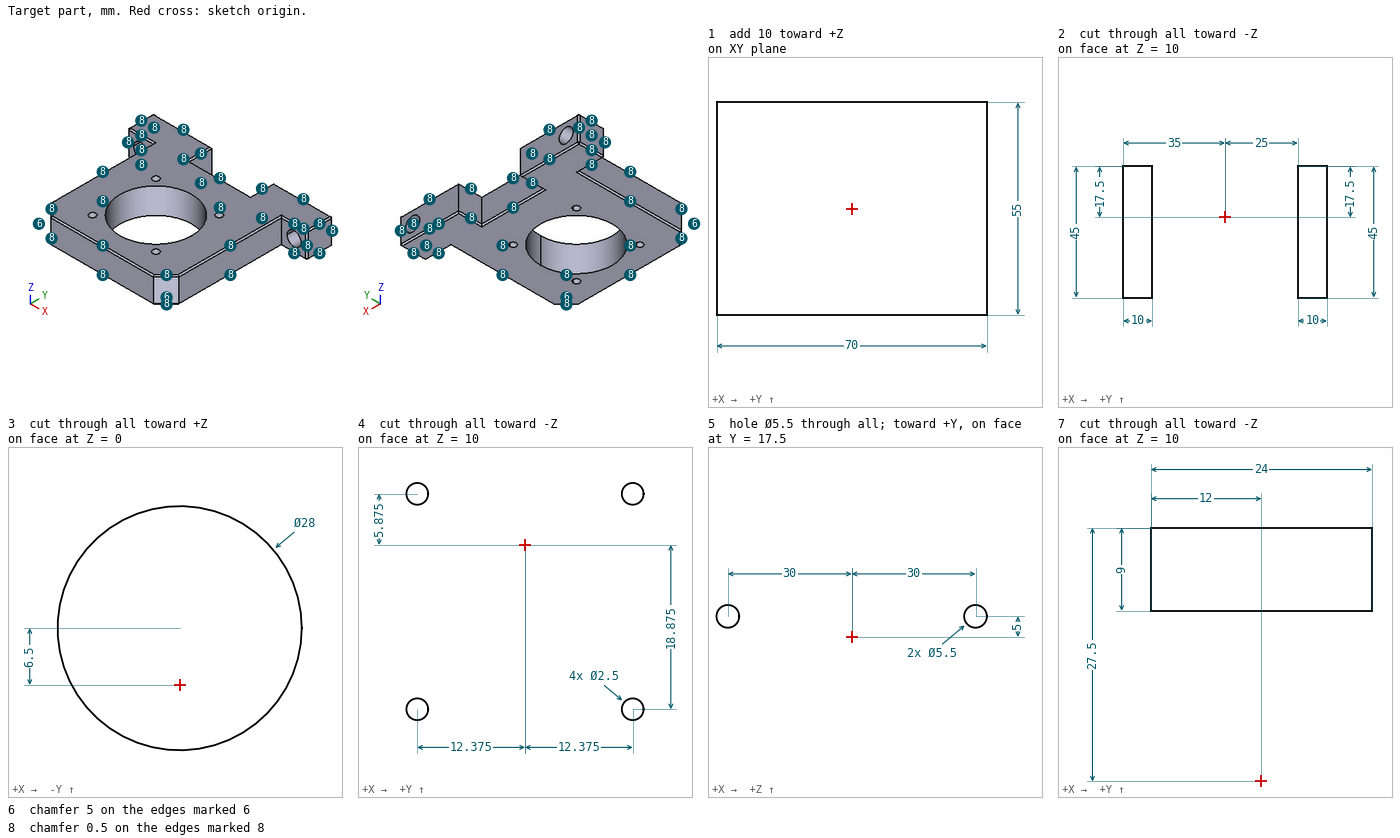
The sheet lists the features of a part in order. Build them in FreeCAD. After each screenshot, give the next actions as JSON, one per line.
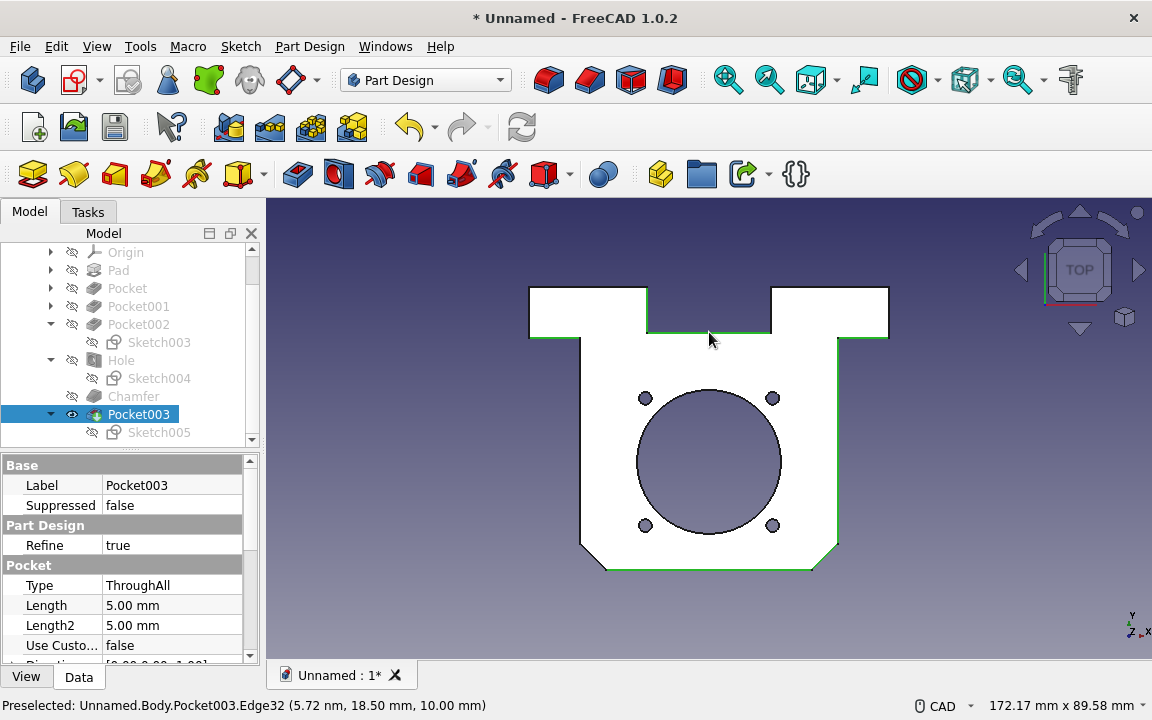
{"action": "left_click", "coordinate": [771, 309], "text": "ctrl"}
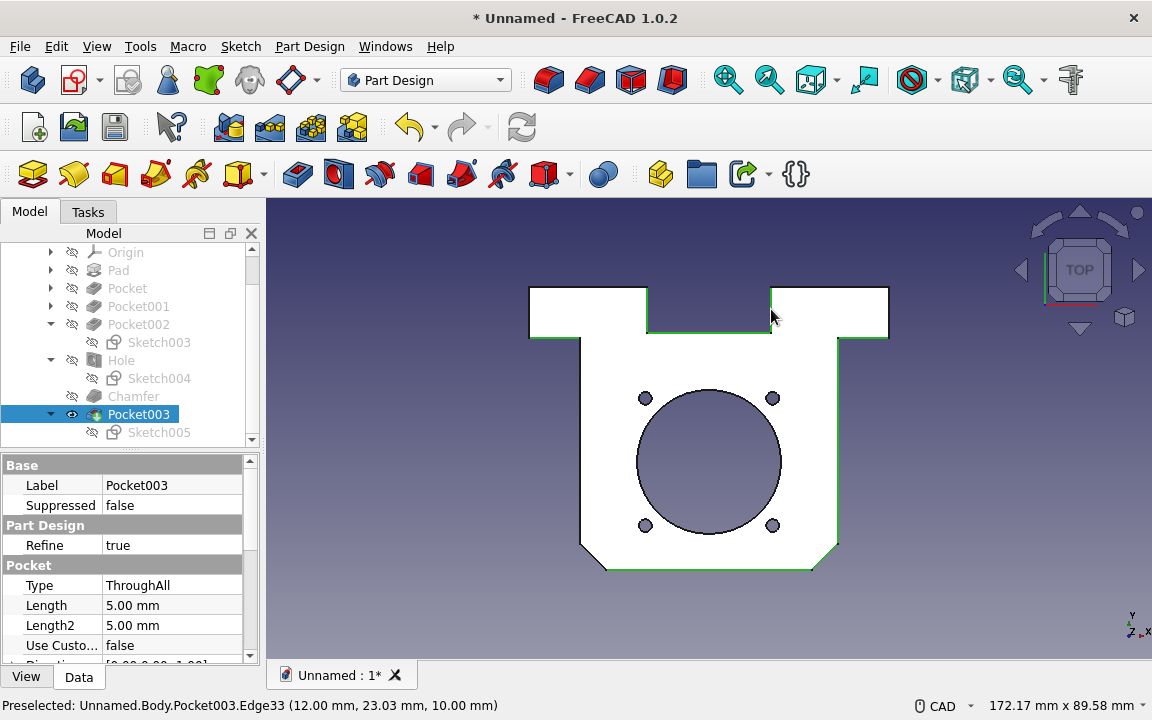
{"action": "left_click", "coordinate": [830, 286], "text": "ctrl"}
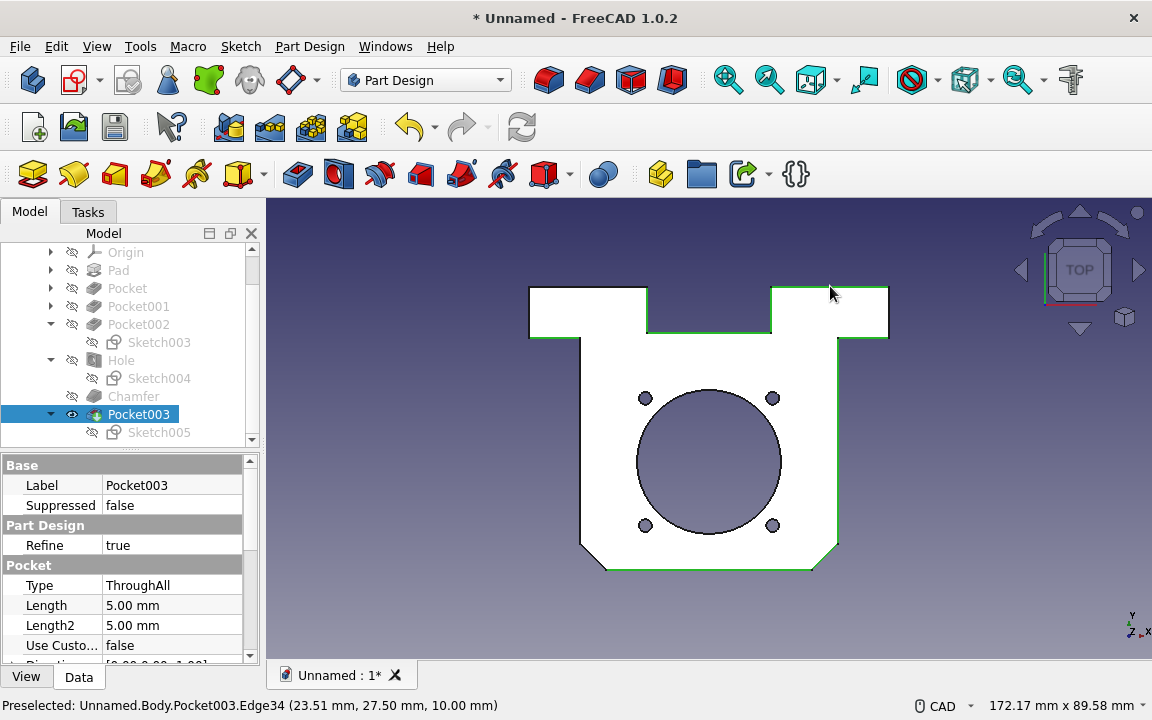
{"action": "left_click", "coordinate": [580, 440], "text": "ctrl"}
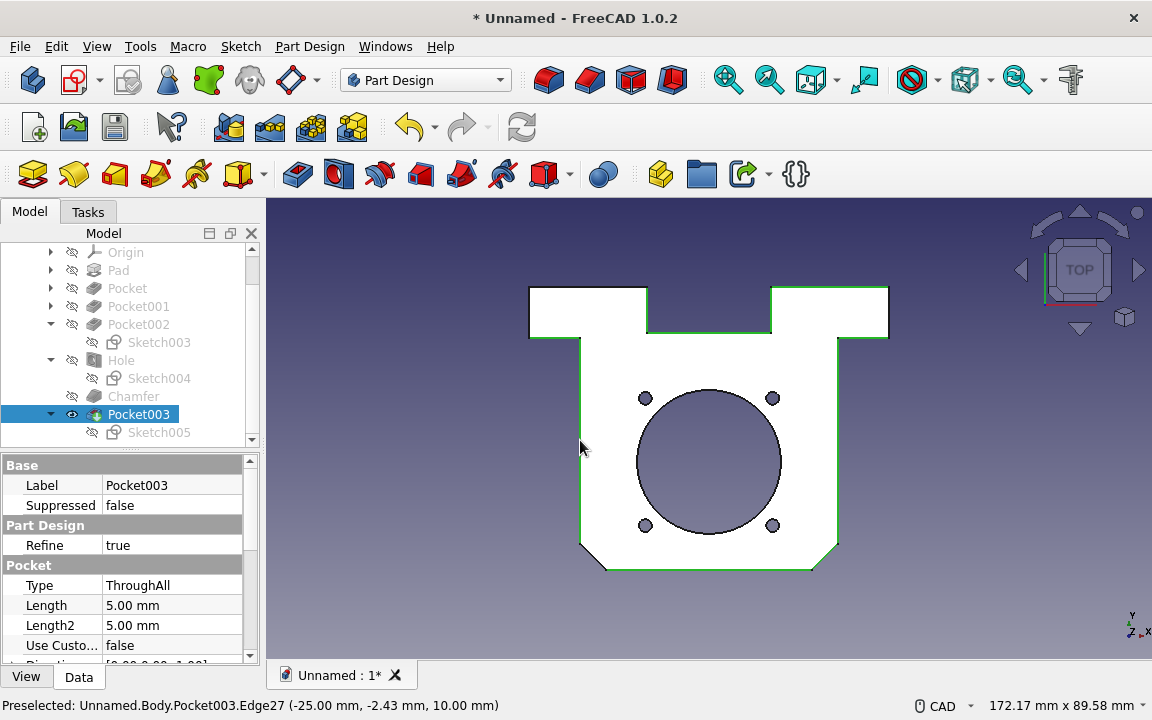
{"action": "left_click", "coordinate": [593, 556], "text": "ctrl"}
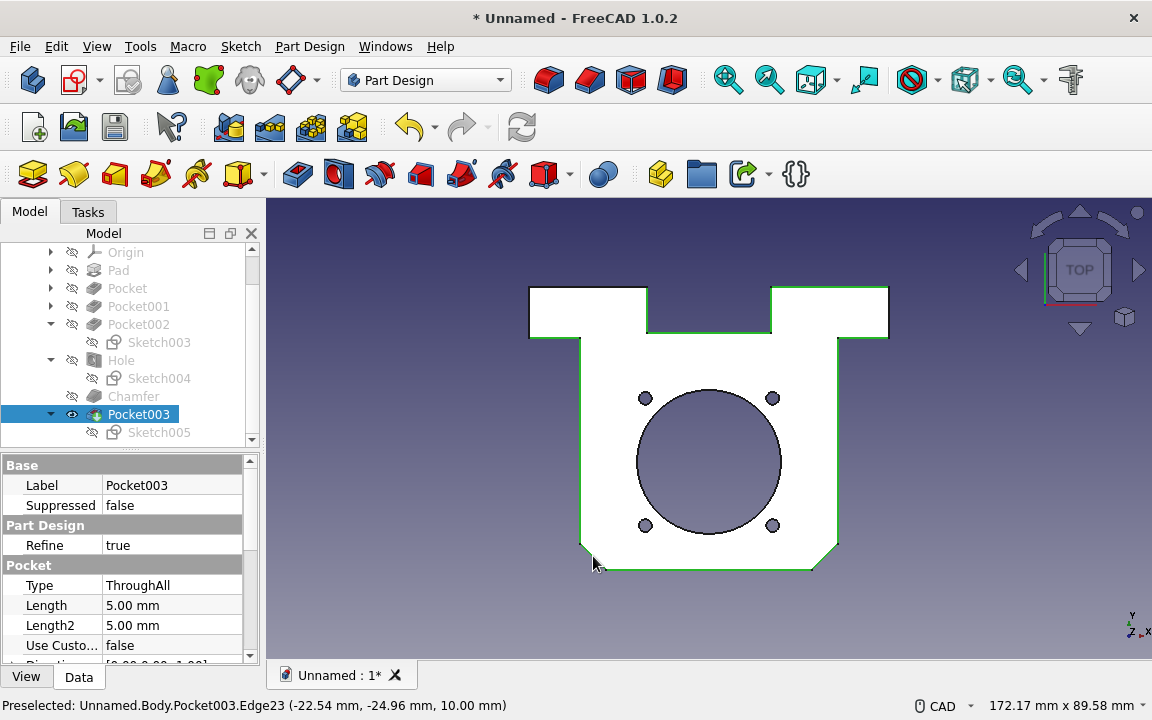
{"action": "left_click", "coordinate": [588, 286], "text": "ctrl"}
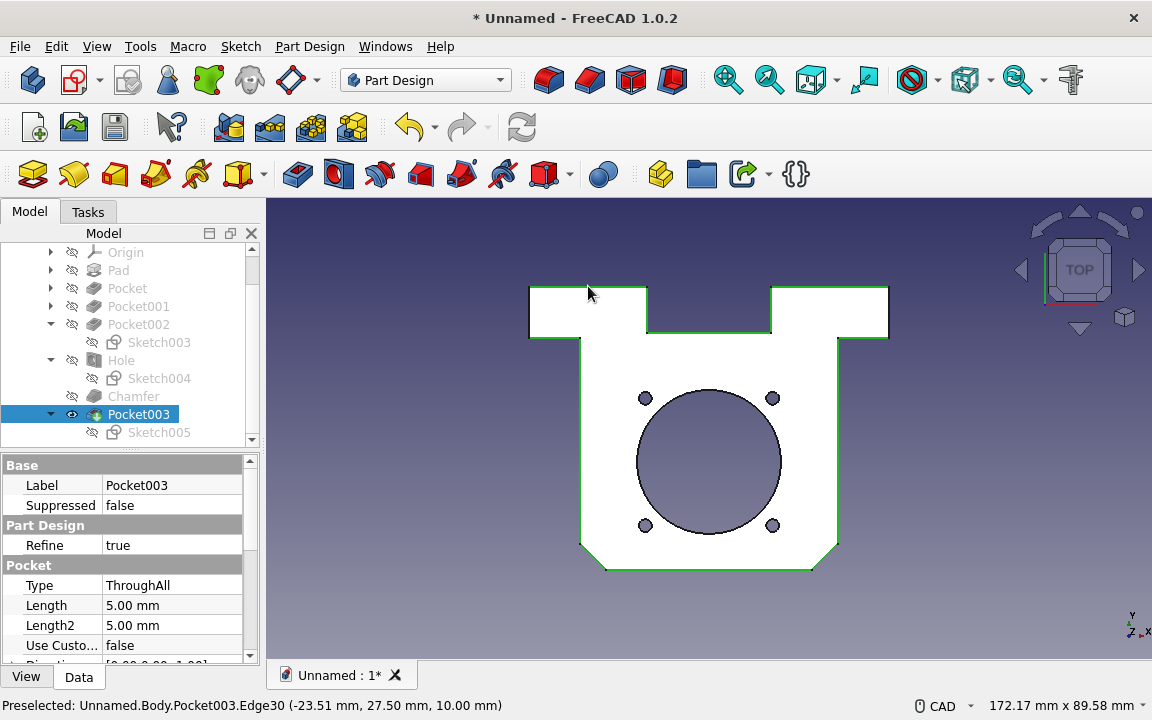
{"action": "key", "text": "0"}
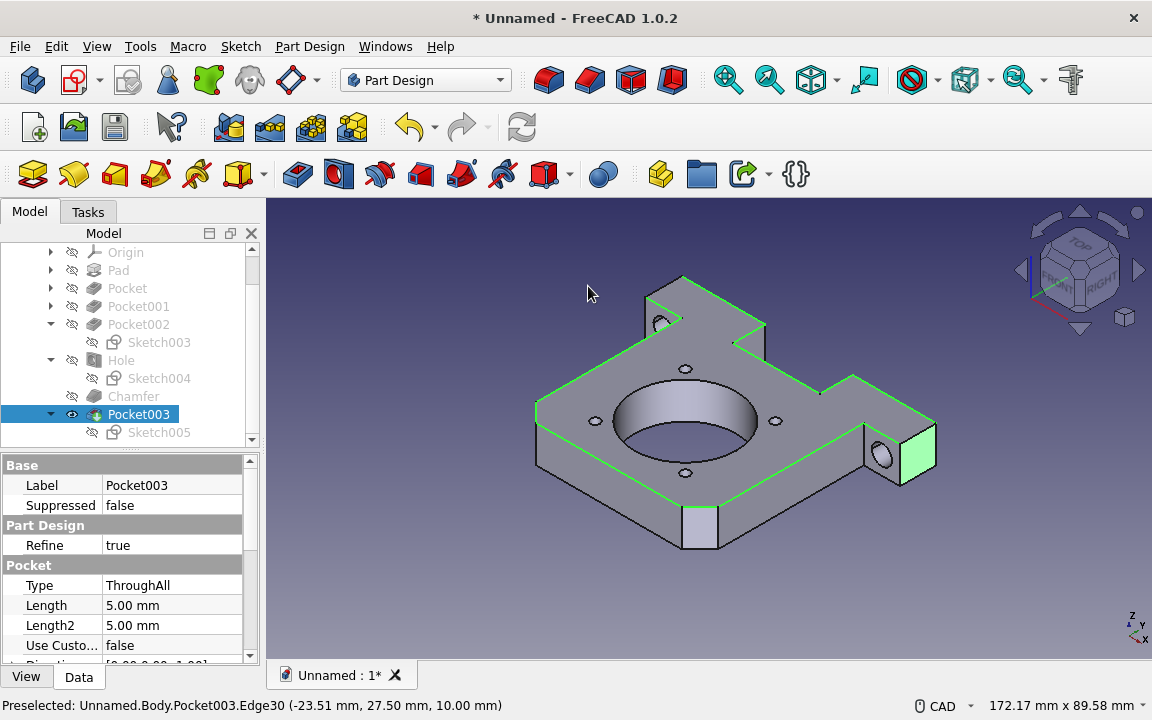
{"action": "key", "text": "1"}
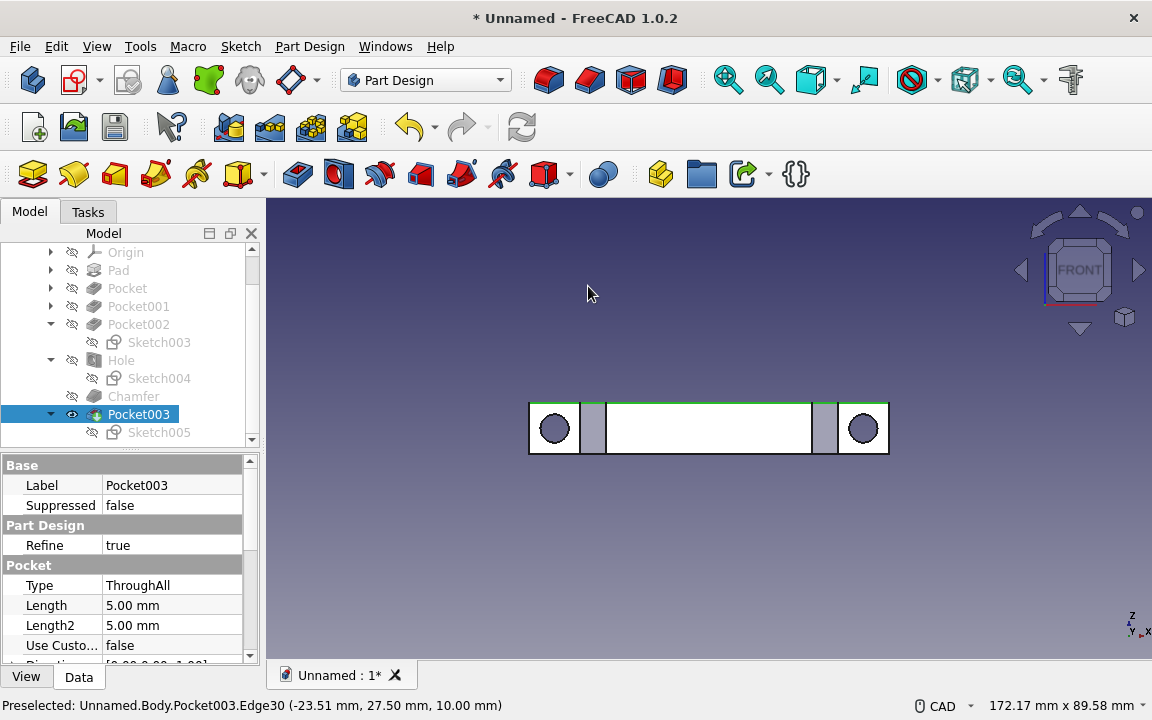
{"action": "left_click", "coordinate": [729, 80]}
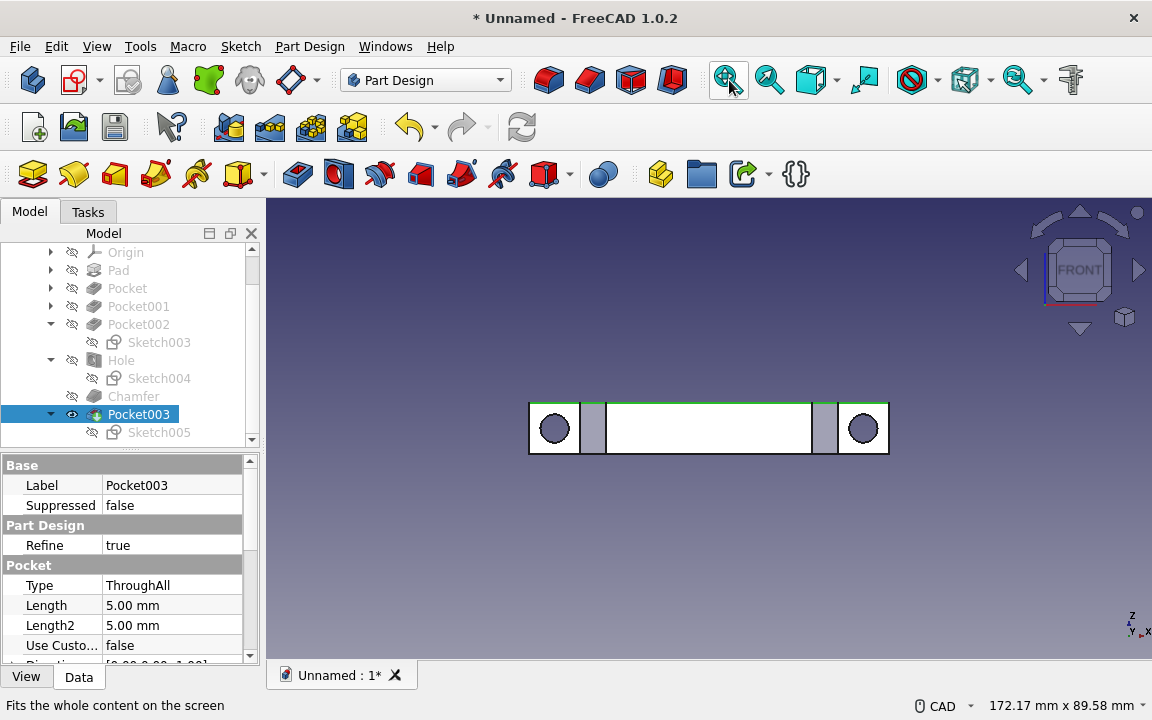
{"action": "left_click", "coordinate": [555, 453], "text": "ctrl"}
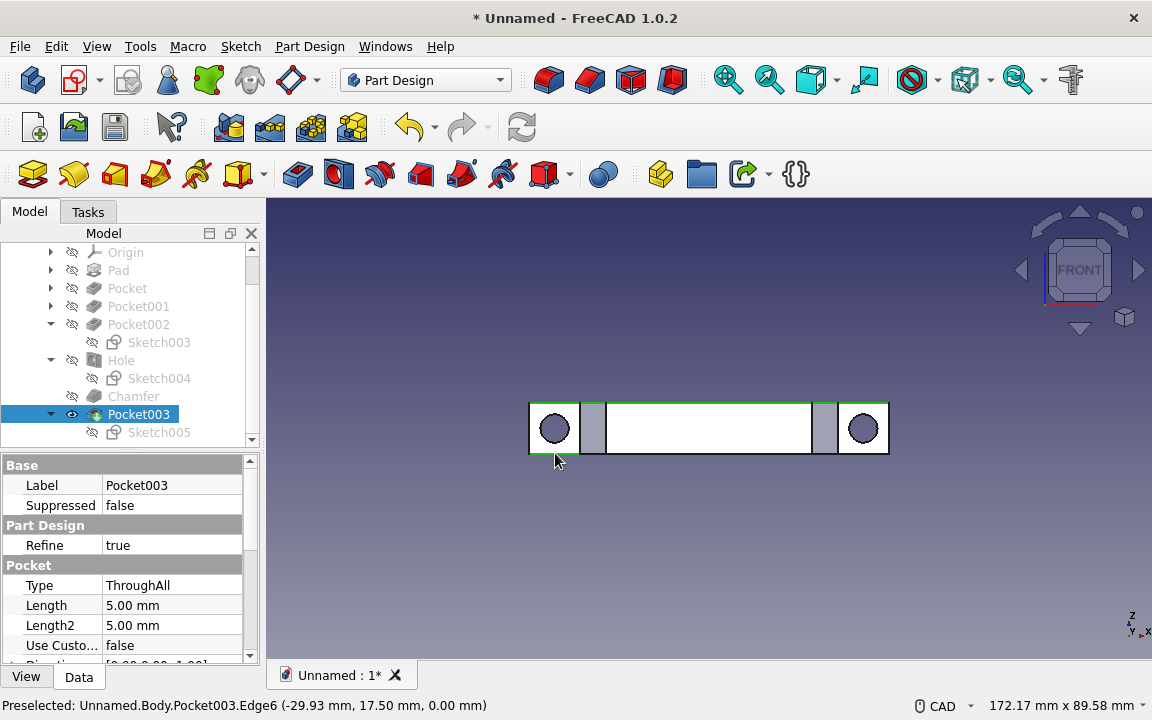
{"action": "left_click", "coordinate": [863, 453], "text": "ctrl"}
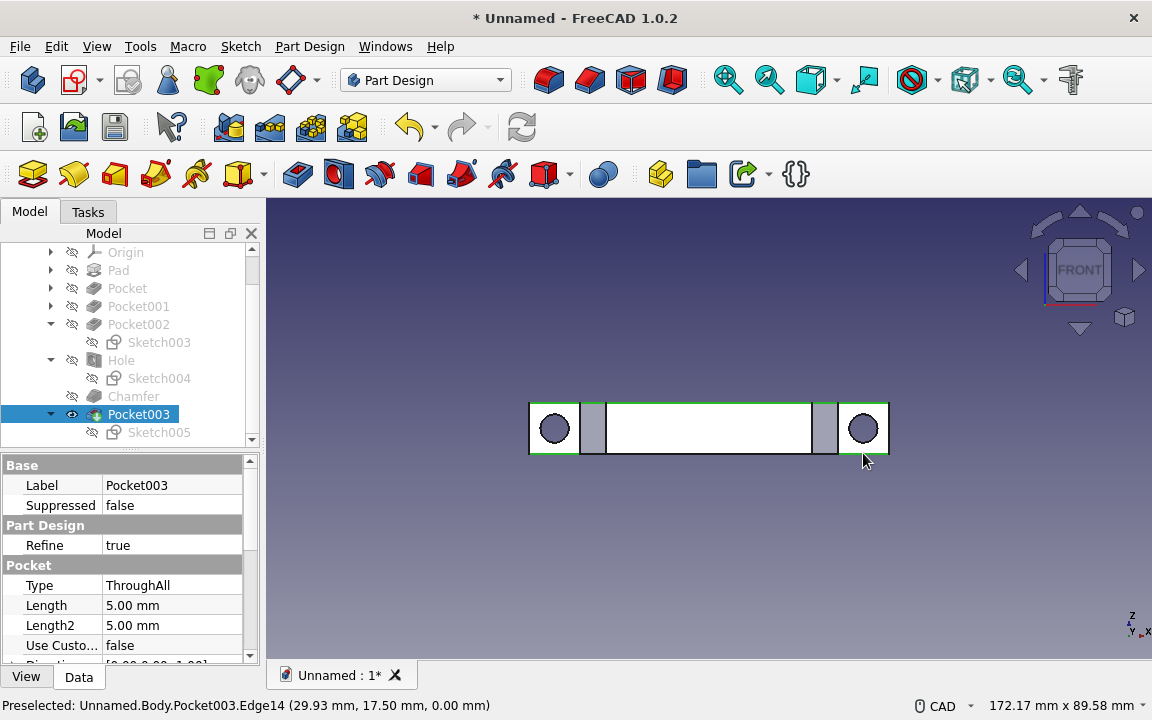
{"action": "left_click", "coordinate": [709, 453], "text": "ctrl"}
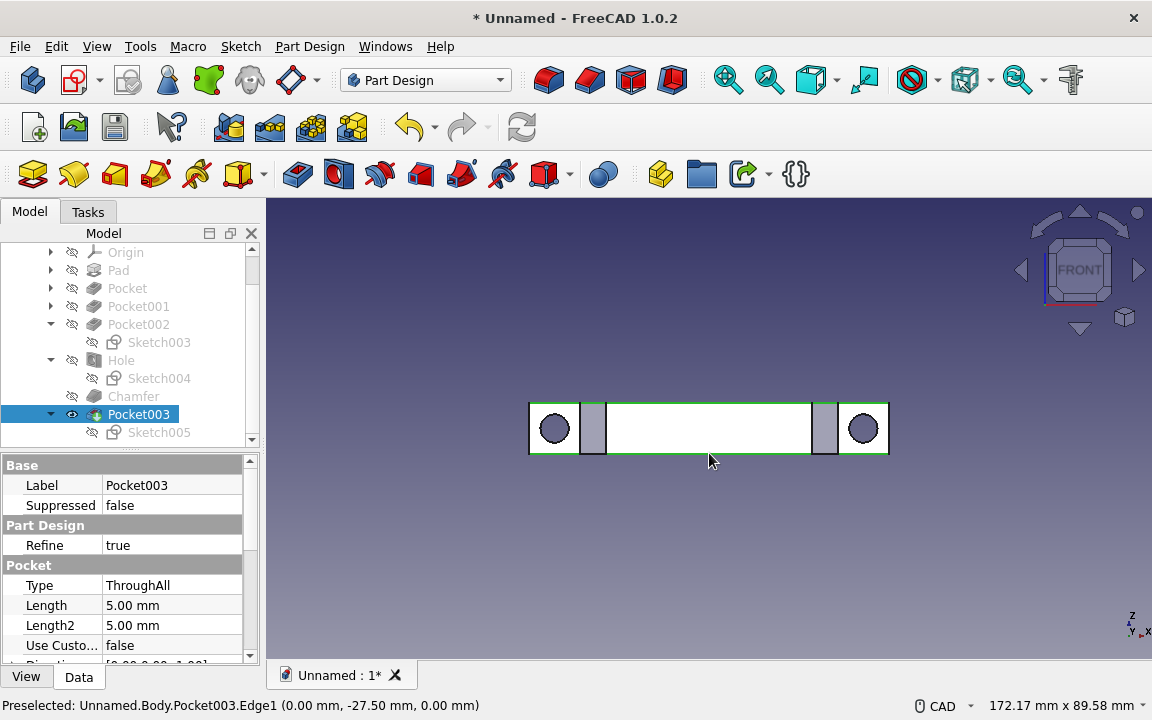
{"action": "left_click", "coordinate": [825, 453], "text": "ctrl"}